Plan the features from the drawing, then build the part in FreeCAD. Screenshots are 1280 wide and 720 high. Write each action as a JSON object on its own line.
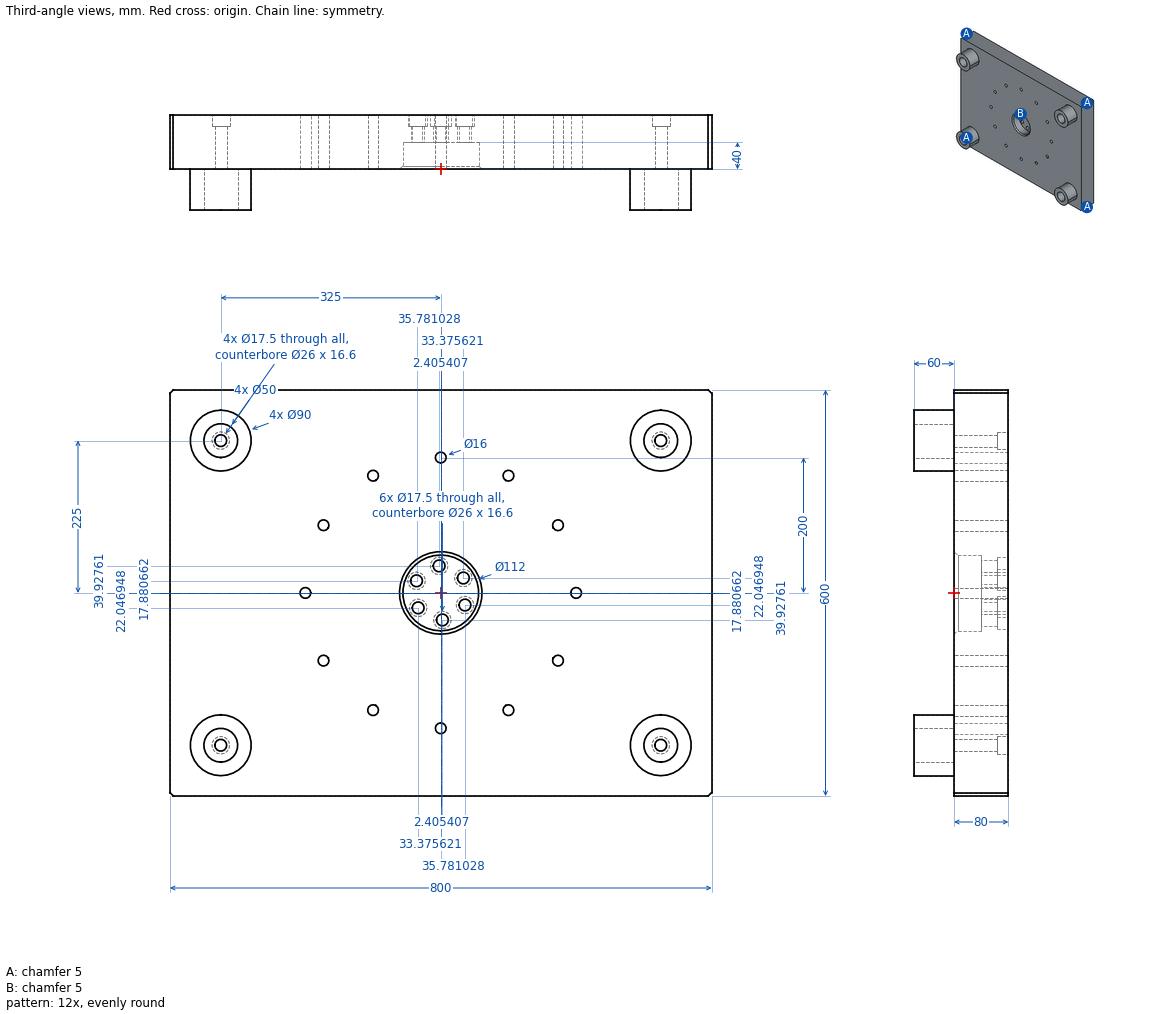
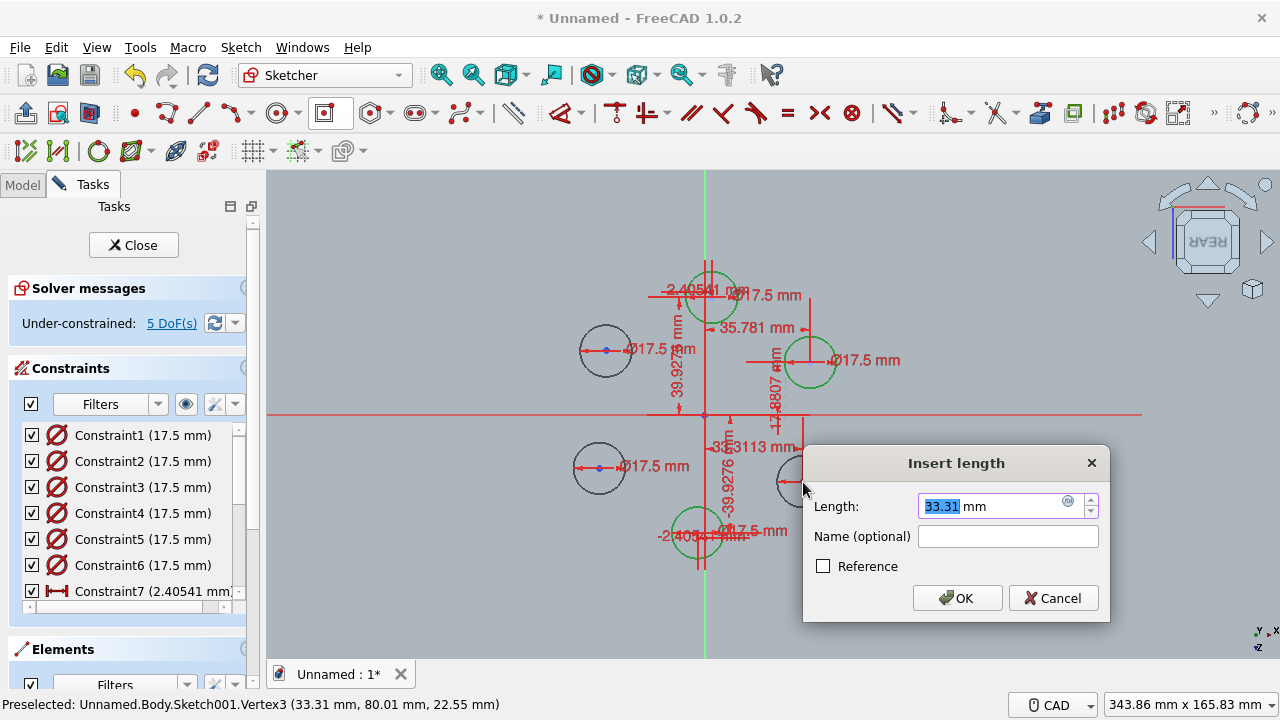
{"action": "type", "text": "33.375621"}
{"action": "key", "text": "Return"}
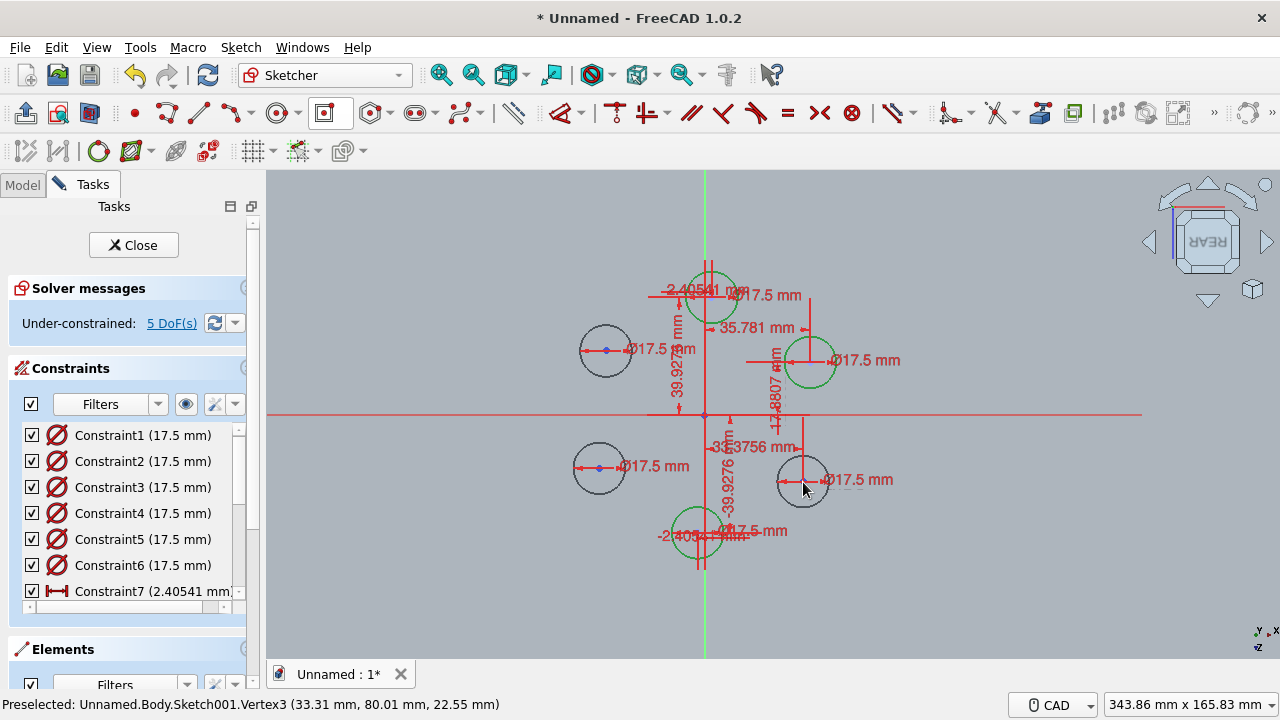
{"action": "left_click", "coordinate": [803, 482]}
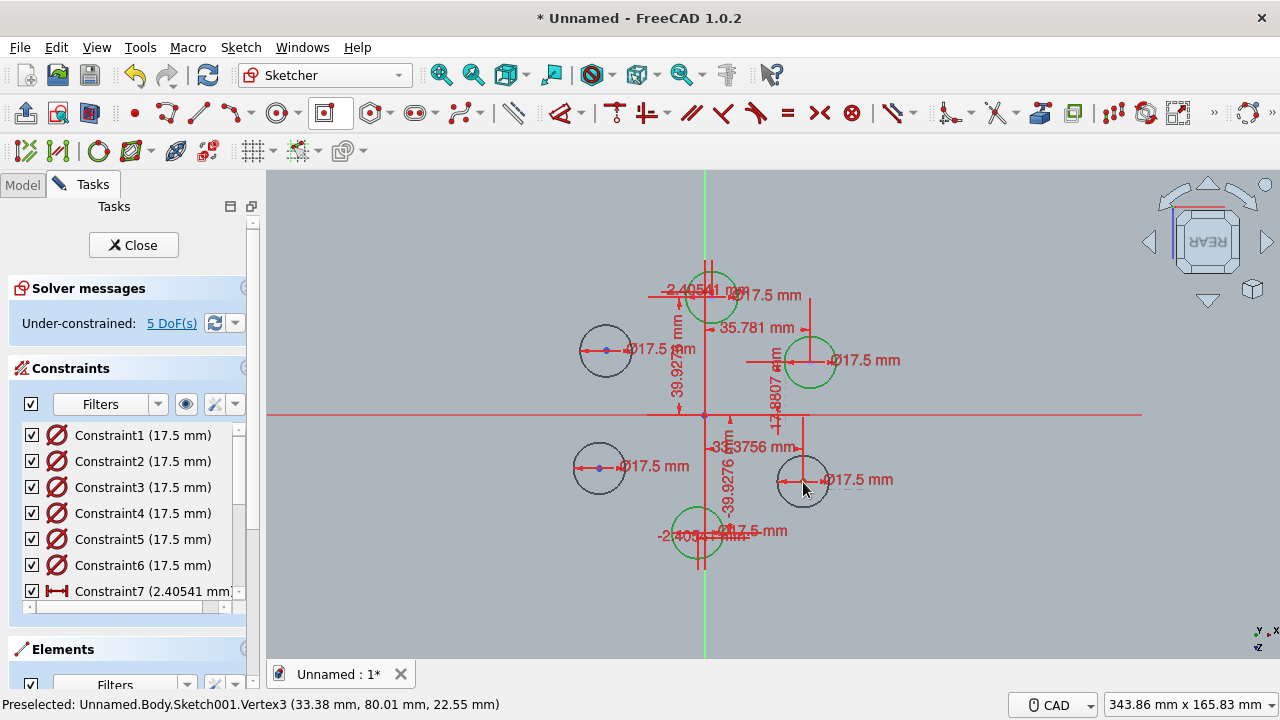
{"action": "key", "text": "i"}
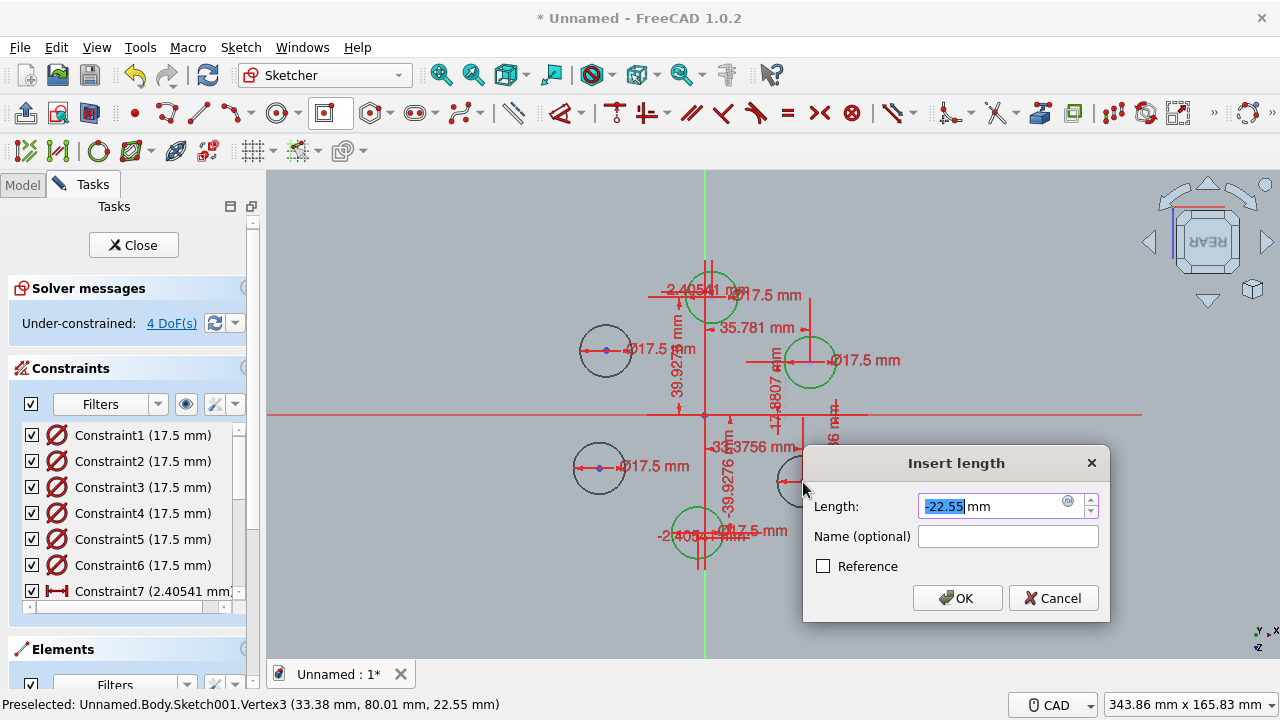
{"action": "type", "text": "-22.046948"}
{"action": "key", "text": "Return"}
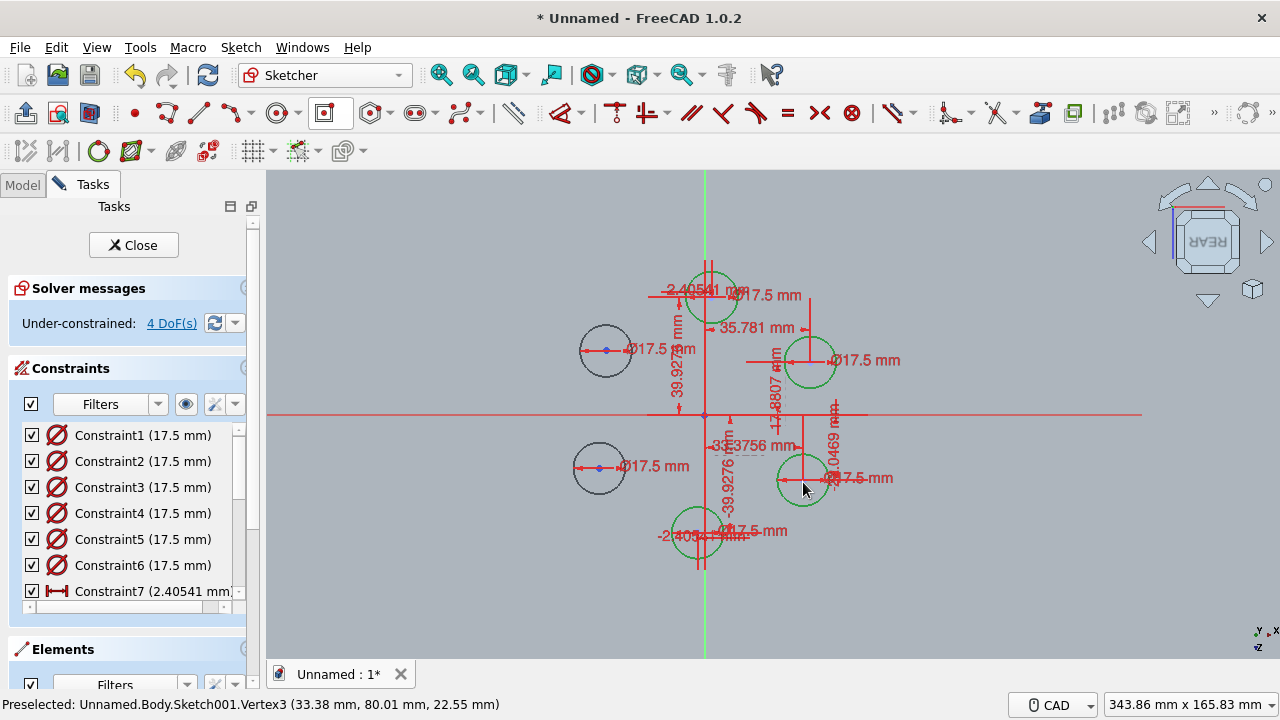
{"action": "left_click", "coordinate": [599, 468]}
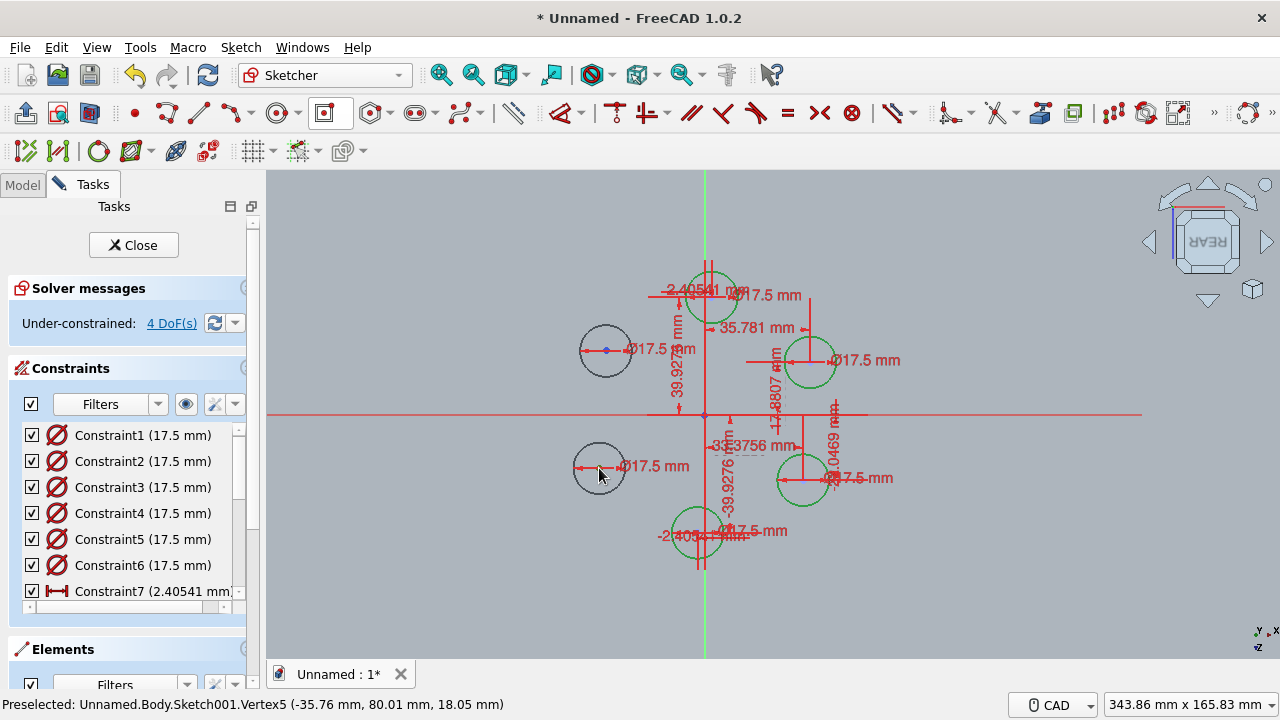
{"action": "key", "text": "l"}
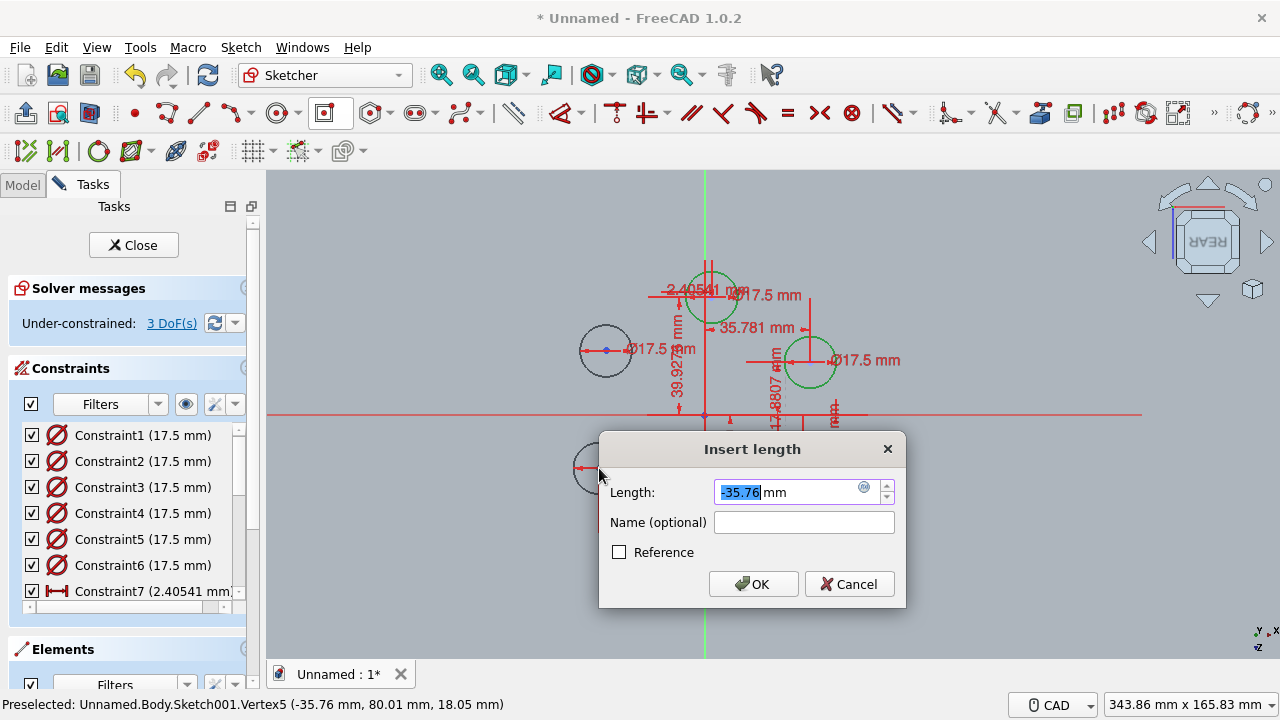
{"action": "type", "text": "-35.781028"}
{"action": "key", "text": "Return"}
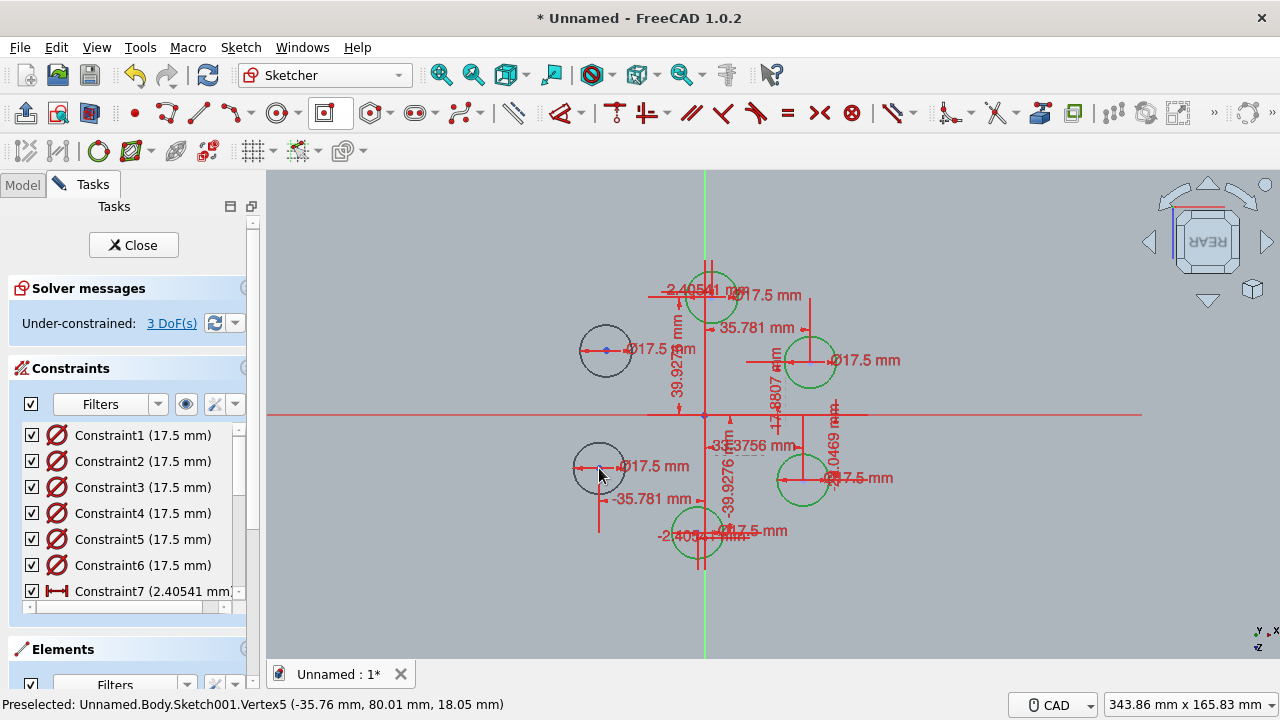
{"action": "left_click", "coordinate": [599, 468]}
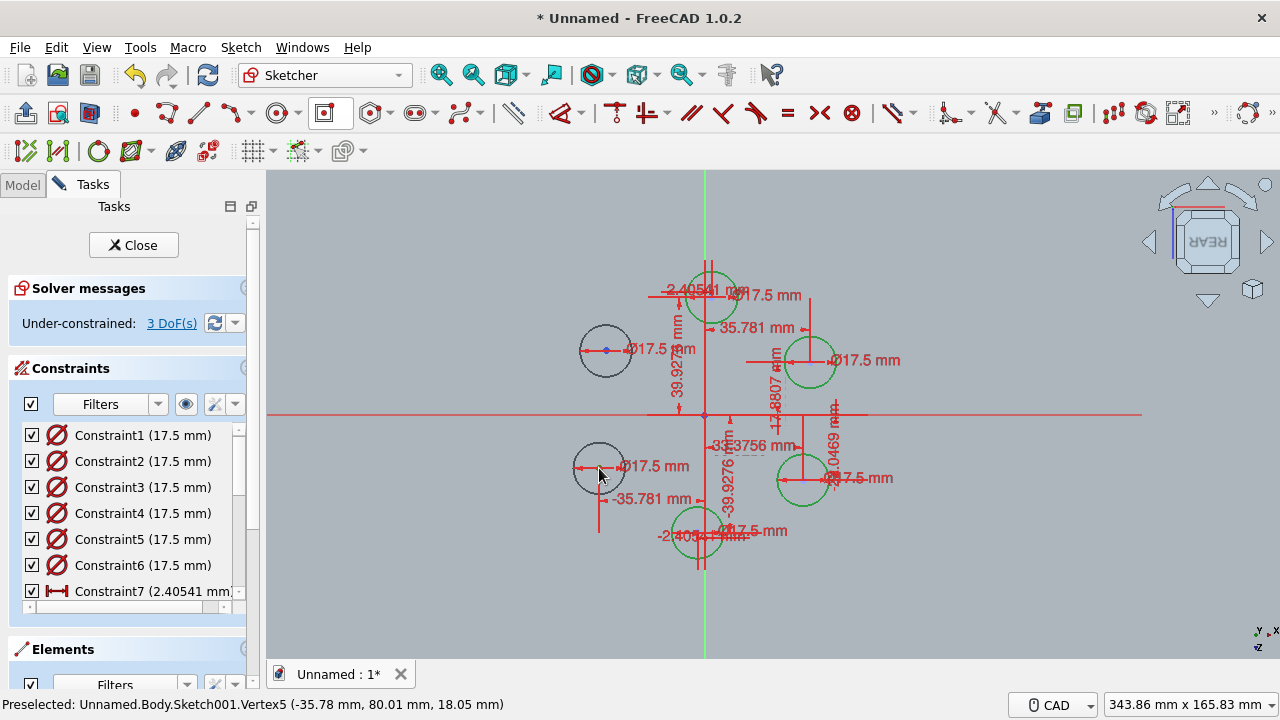
{"action": "key", "text": "i"}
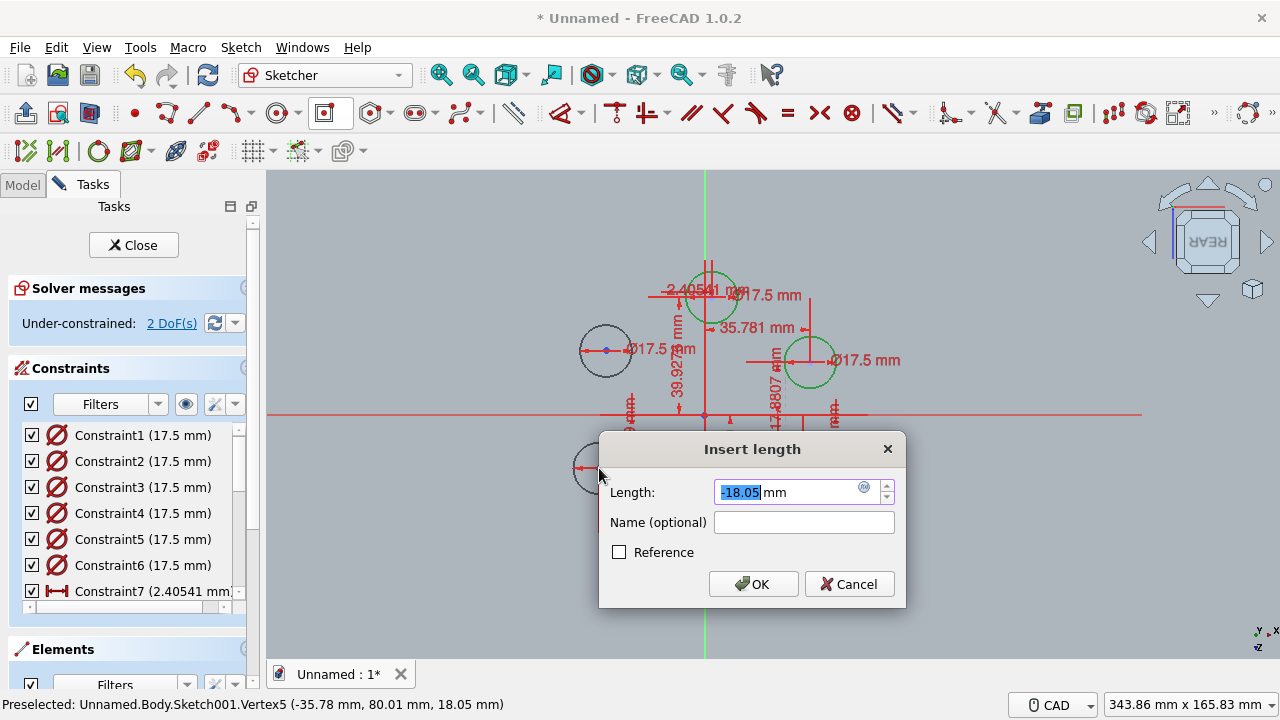
{"action": "type", "text": "-17.880662"}
{"action": "key", "text": "Return"}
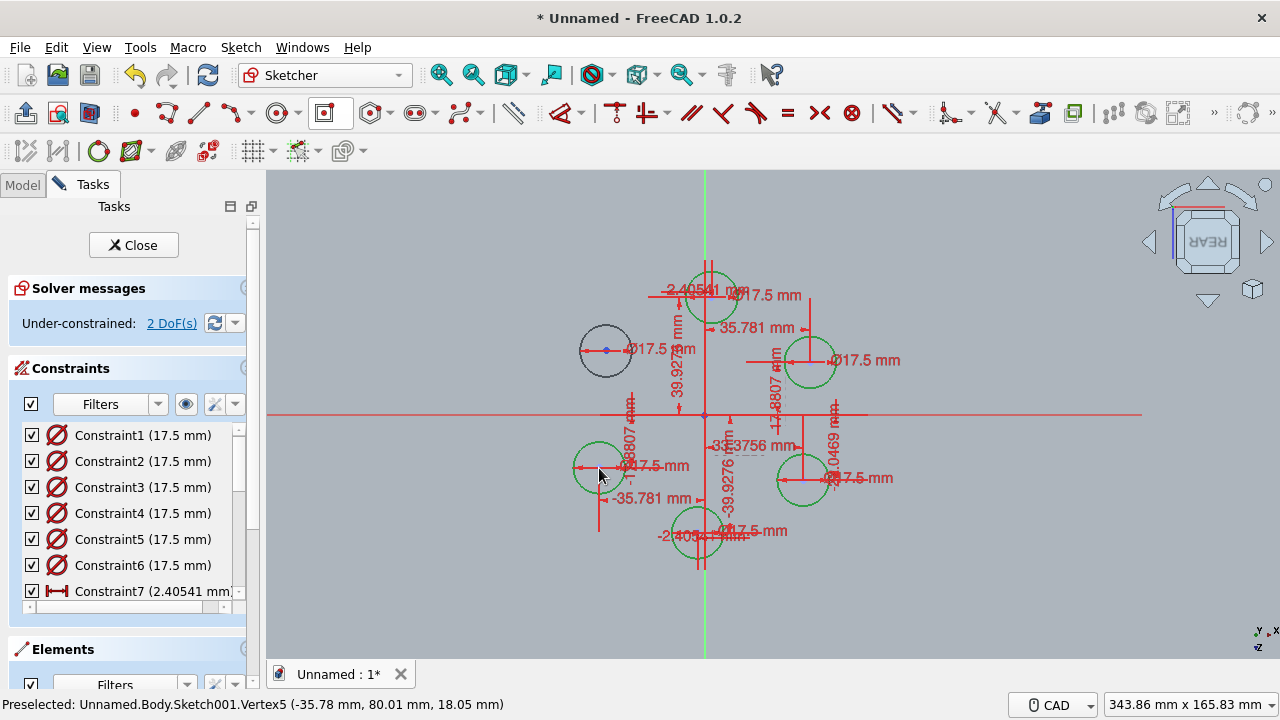
{"action": "left_click", "coordinate": [606, 351]}